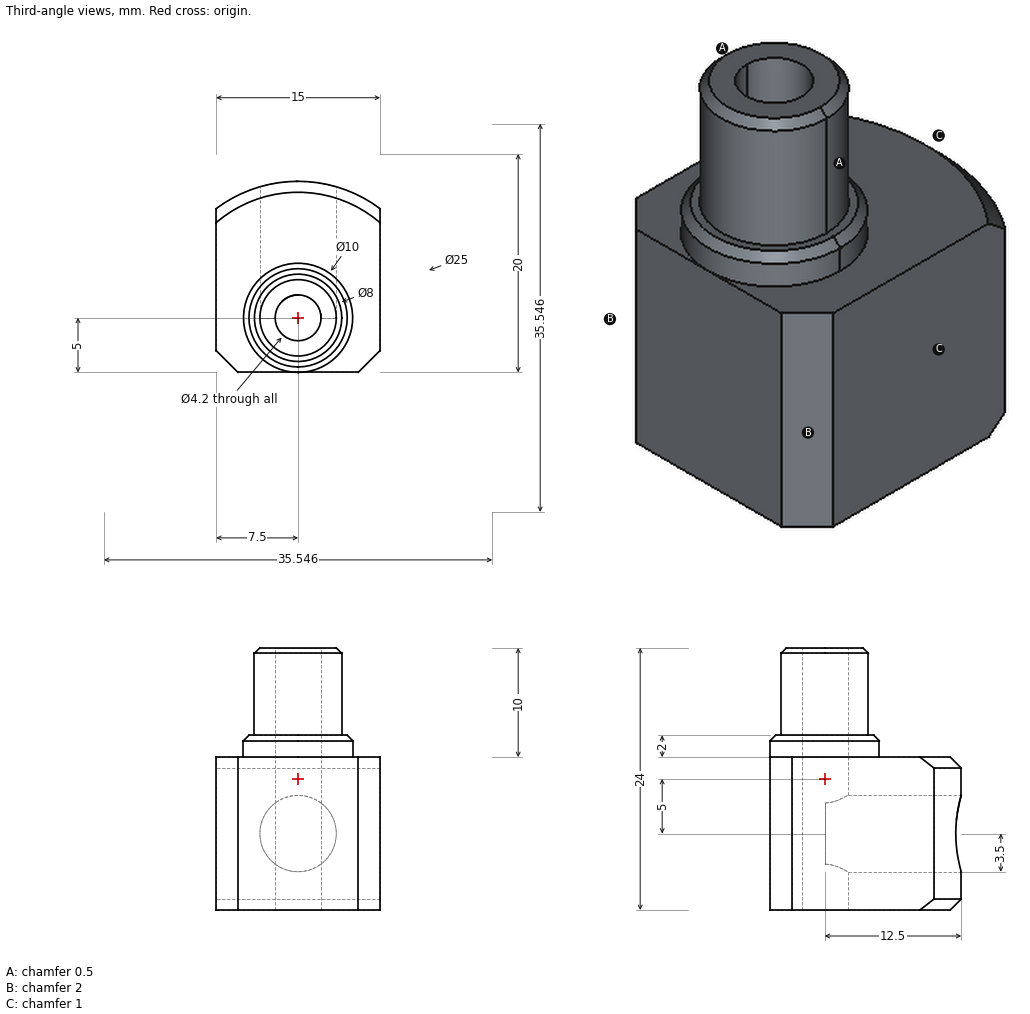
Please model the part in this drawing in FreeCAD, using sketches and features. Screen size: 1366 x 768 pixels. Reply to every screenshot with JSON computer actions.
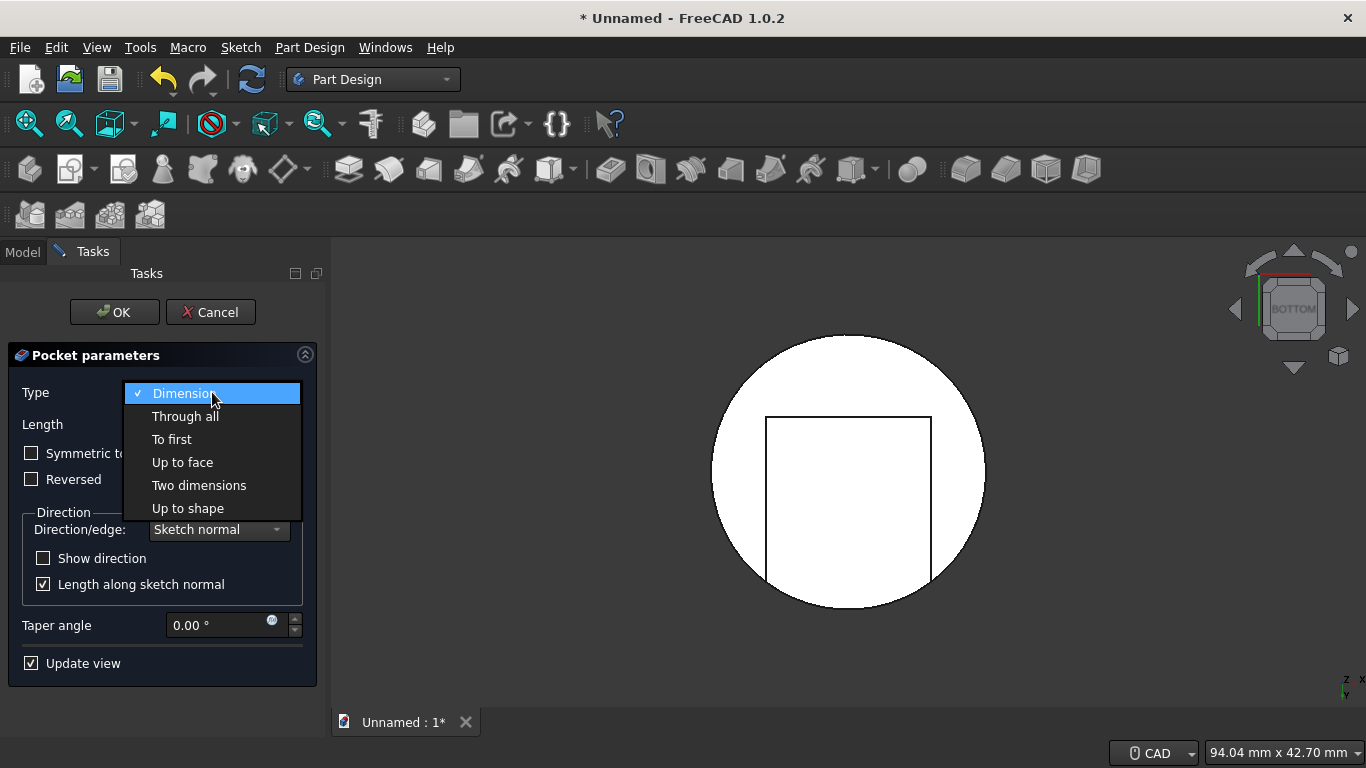
{"action": "left_click", "coordinate": [212, 416]}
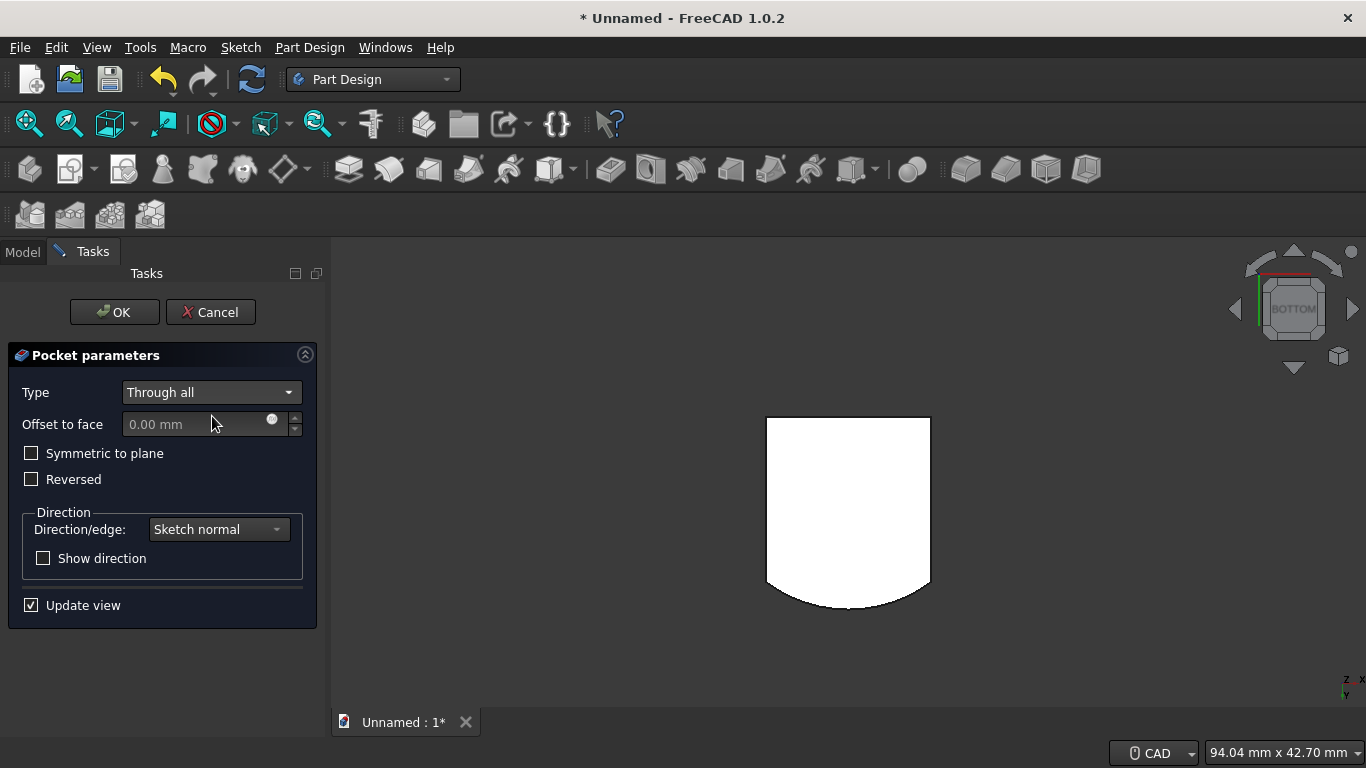
{"action": "left_click", "coordinate": [115, 312]}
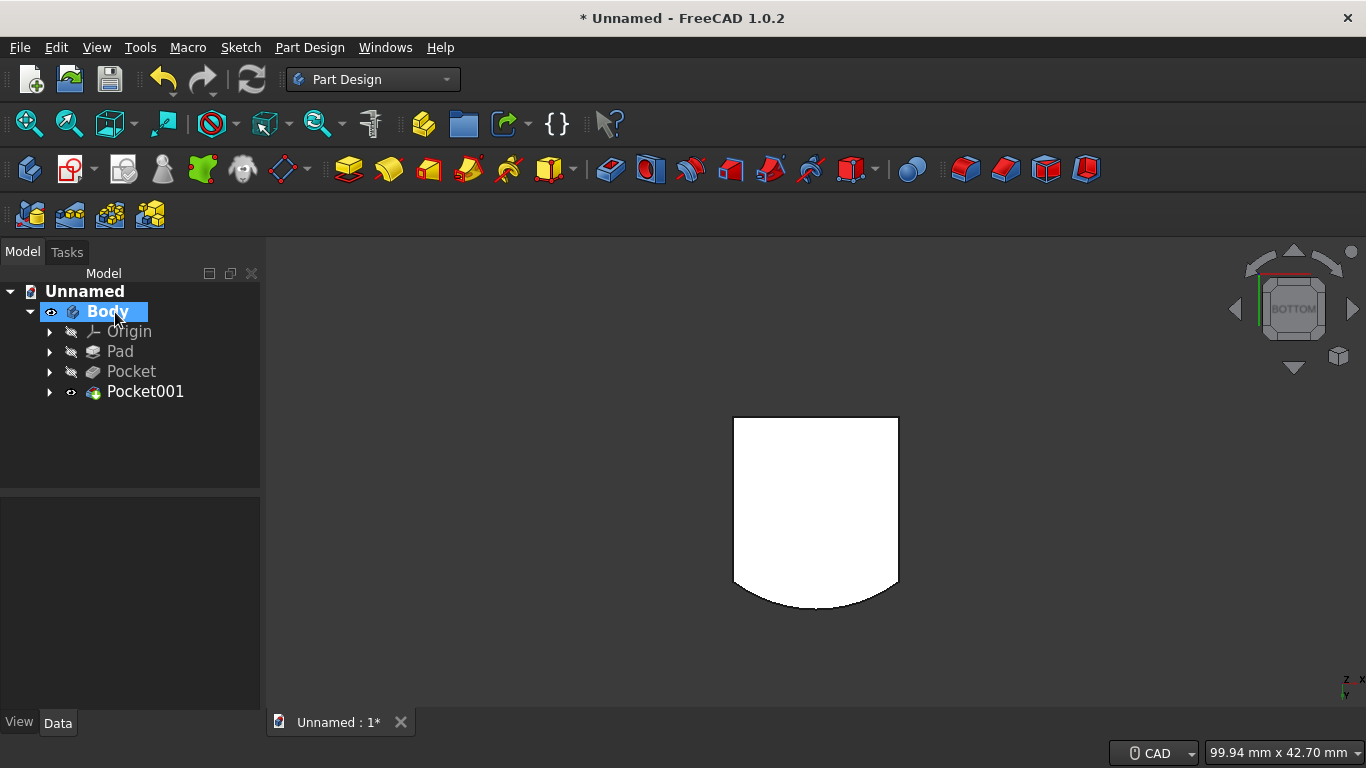
{"action": "left_click", "coordinate": [30, 124]}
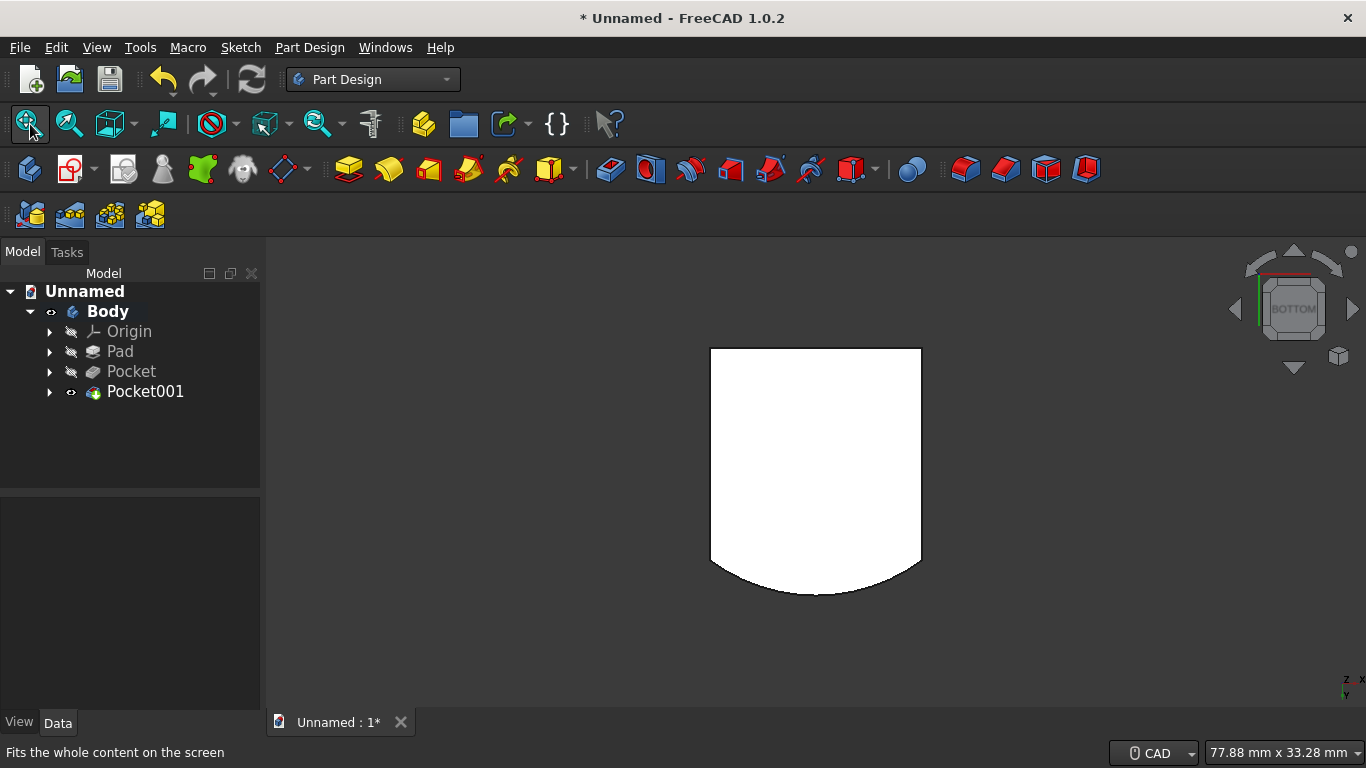
{"action": "left_click", "coordinate": [816, 471]}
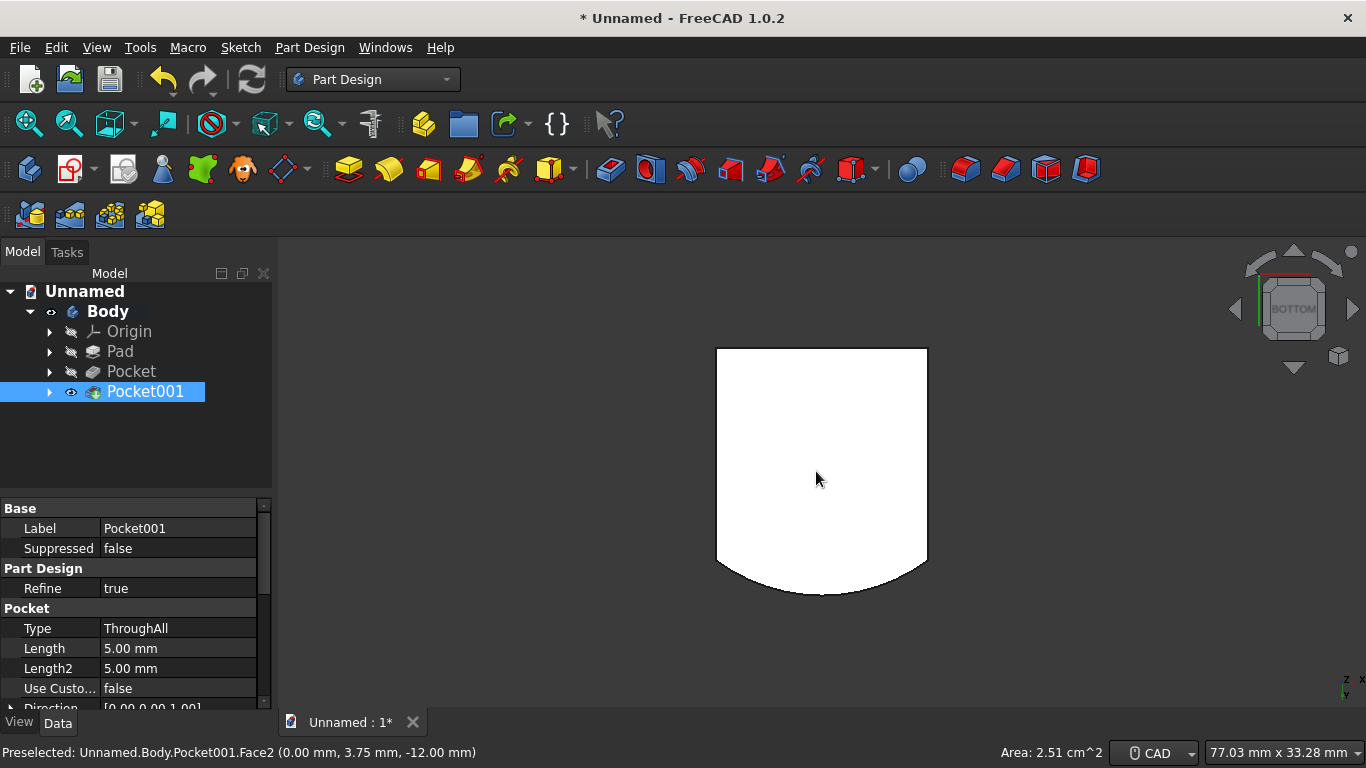
{"action": "left_click", "coordinate": [70, 170]}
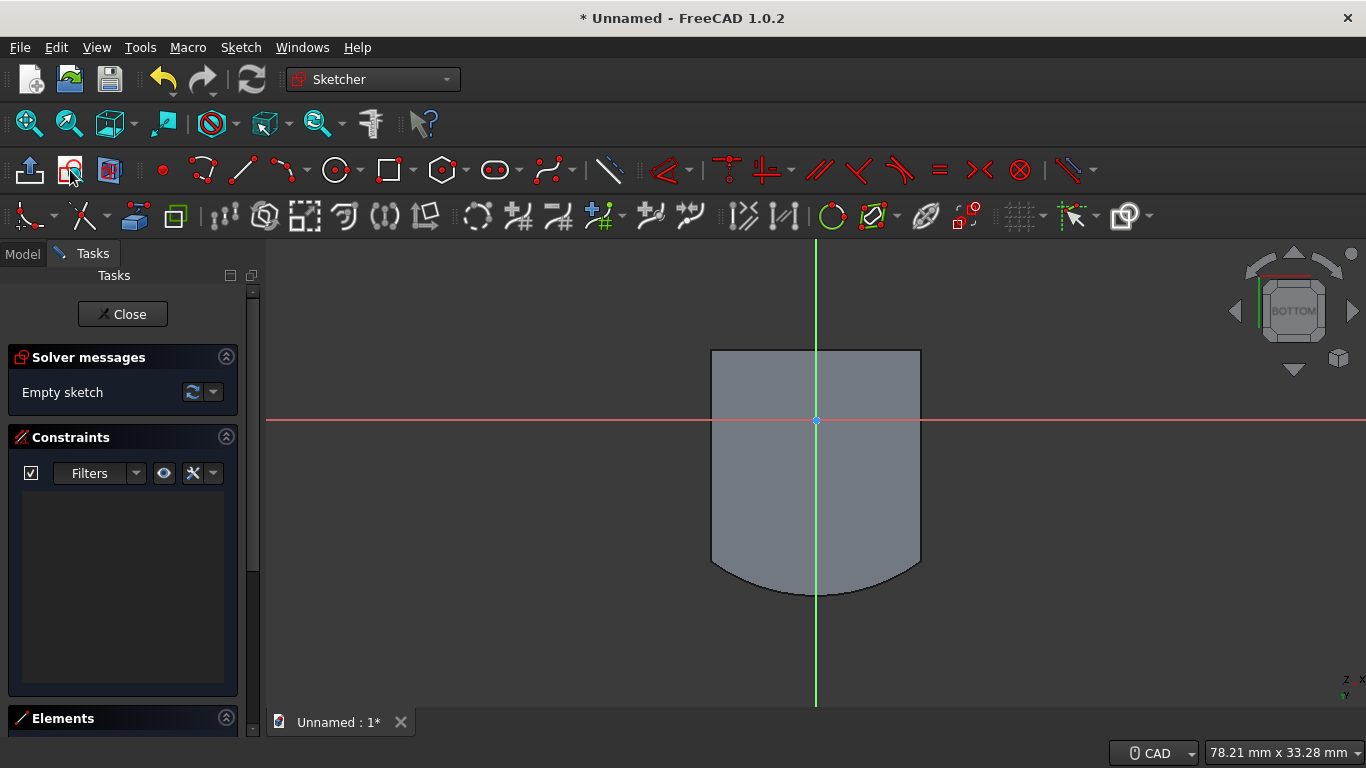
{"action": "scroll", "coordinate": [833, 407], "scroll_direction": "up", "scroll_amount": 8}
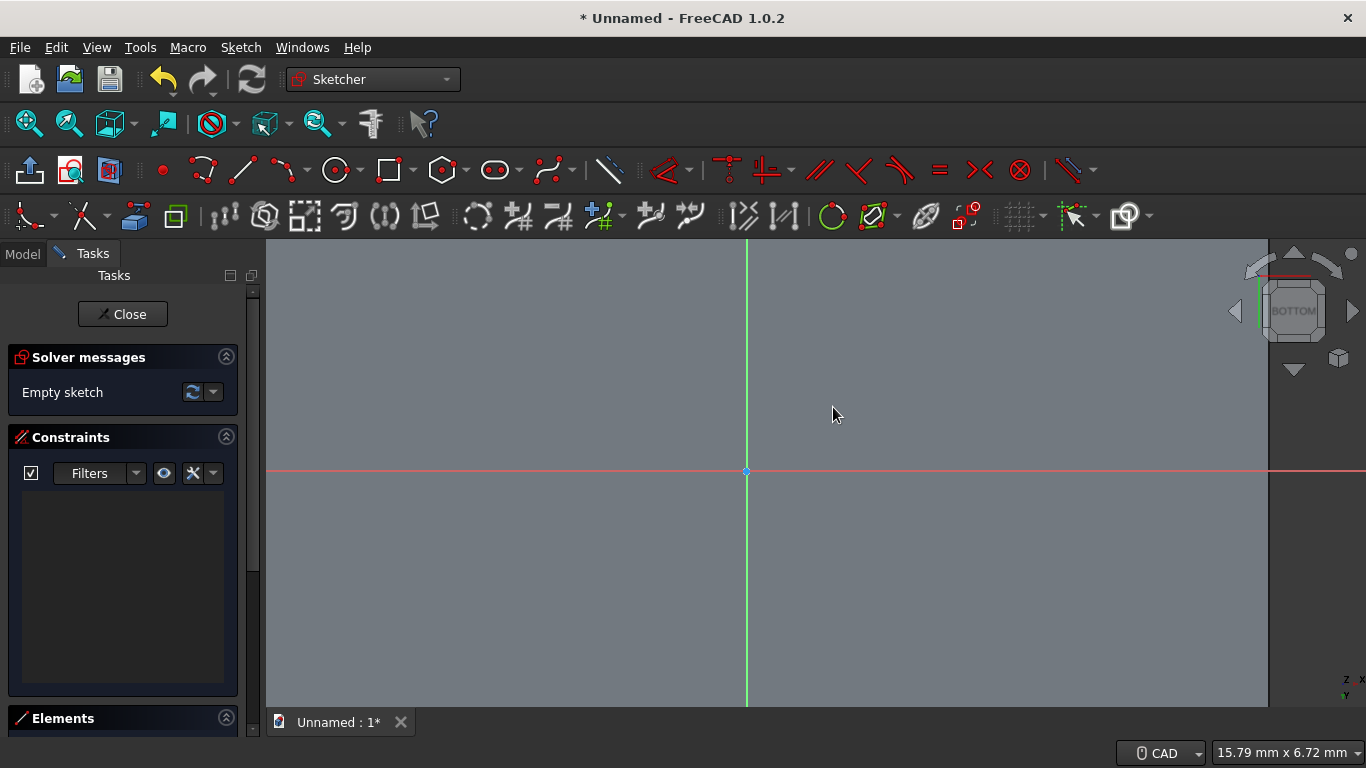
{"action": "left_click", "coordinate": [336, 170]}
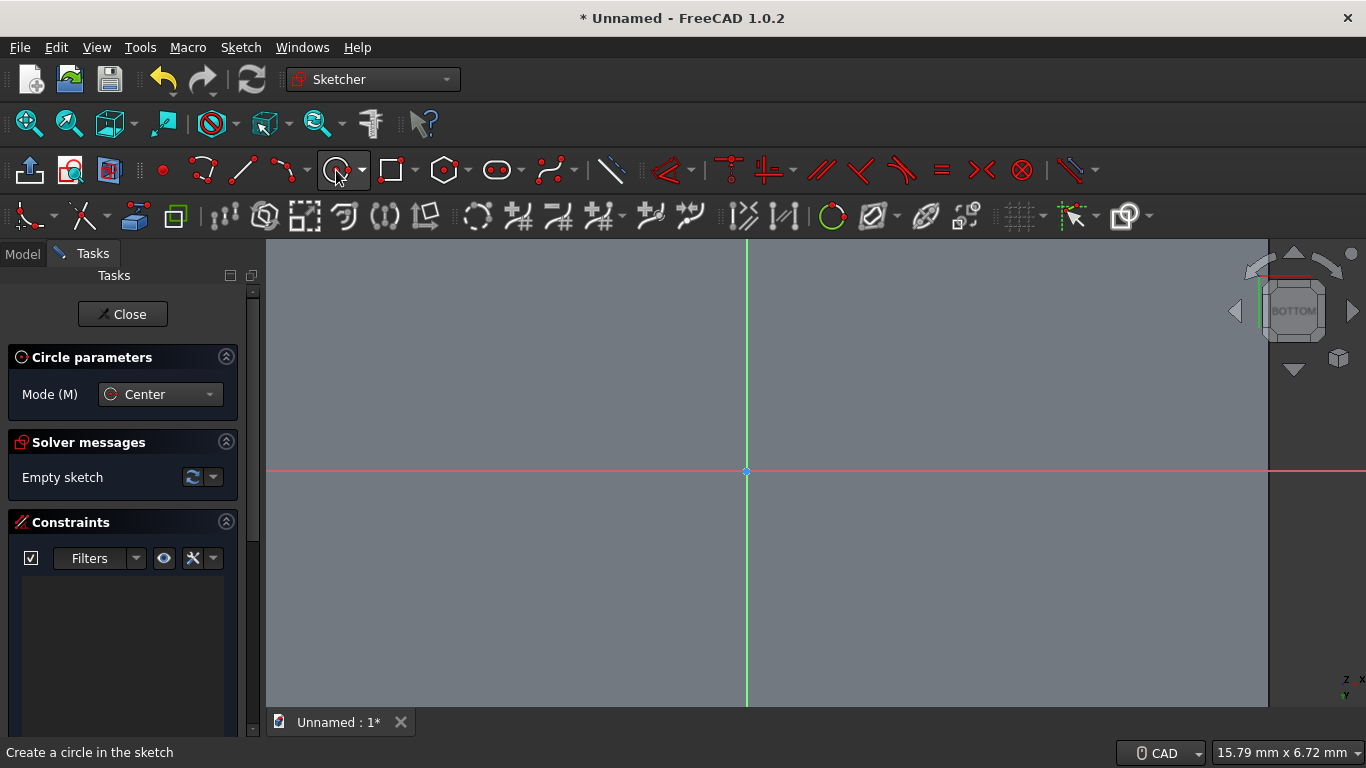
{"action": "left_click", "coordinate": [747, 471]}
{"action": "mouse_move", "coordinate": [850, 368]}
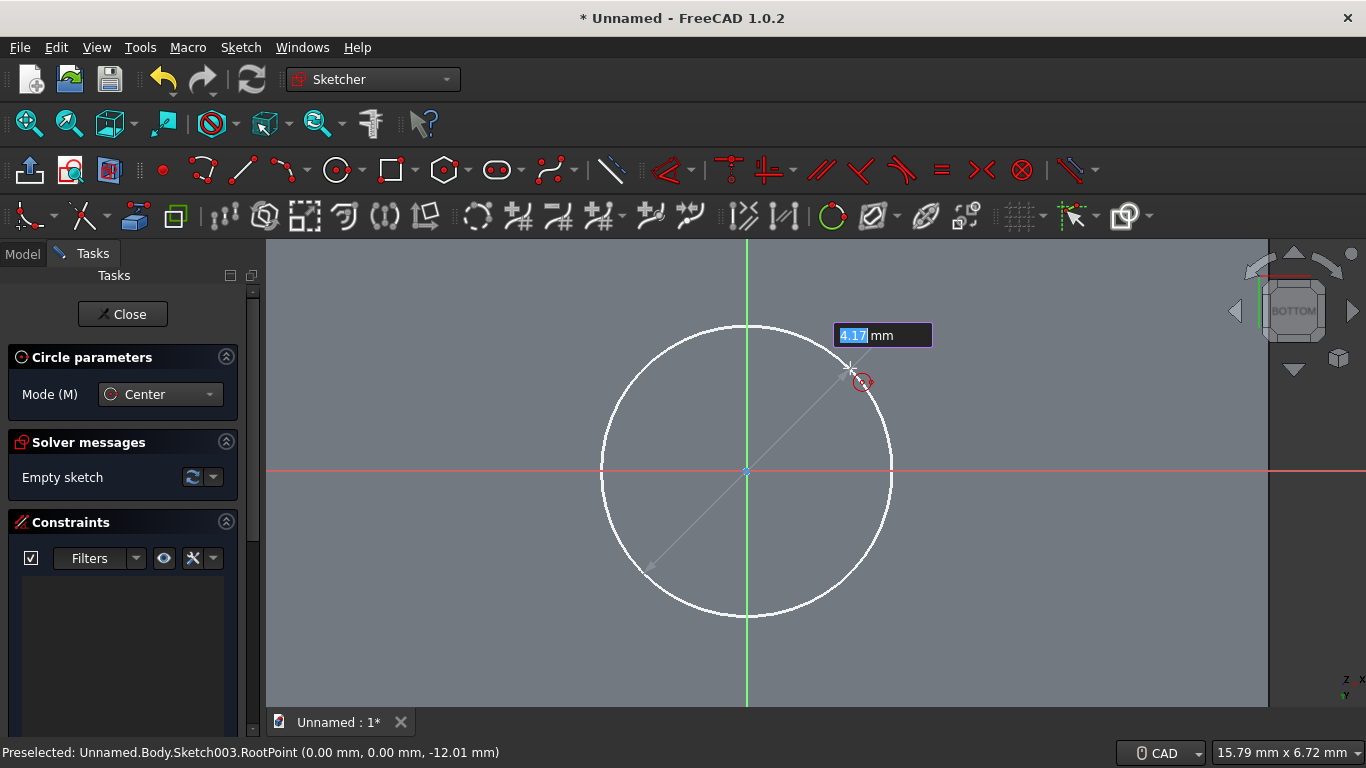
{"action": "type", "text": "4.2"}
{"action": "key", "text": "Return"}
{"action": "key", "text": "Escape"}